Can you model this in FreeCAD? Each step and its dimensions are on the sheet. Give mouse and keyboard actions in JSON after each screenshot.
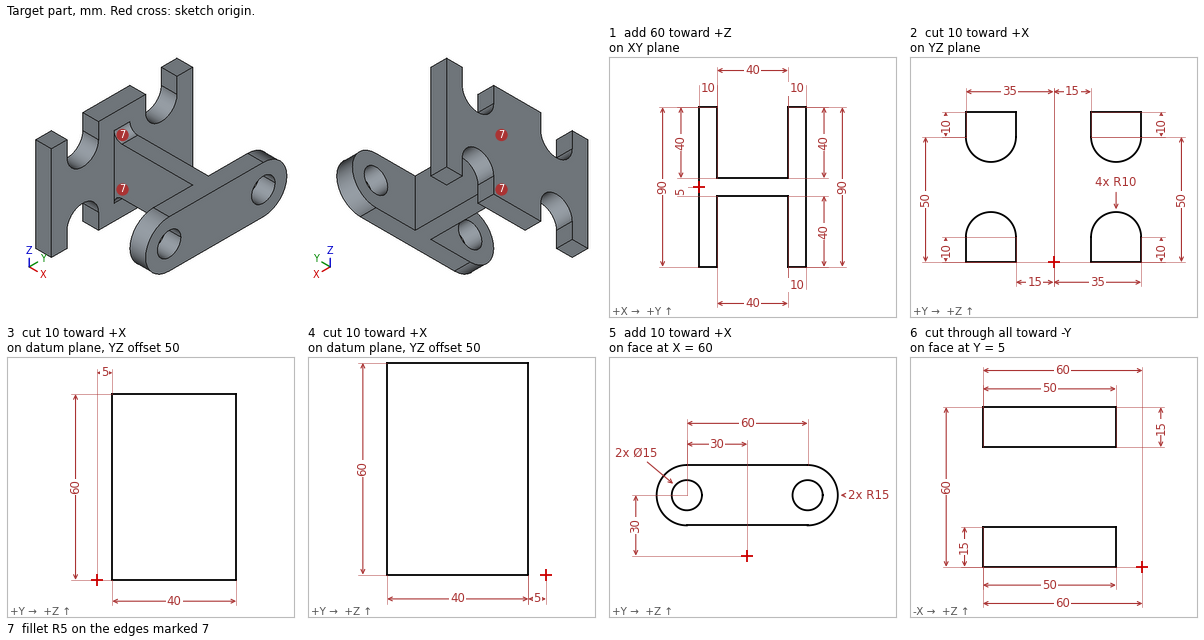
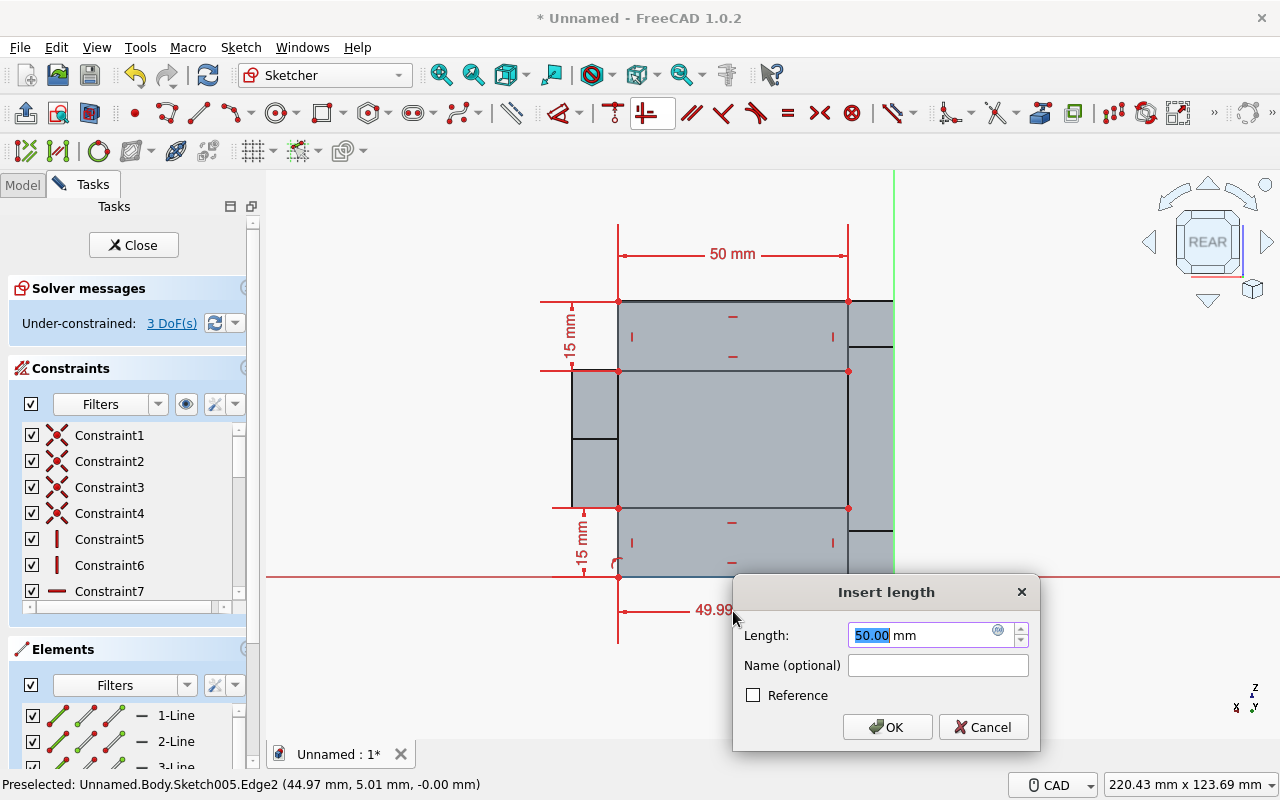
{"action": "type", "text": "50"}
{"action": "key", "text": "Return"}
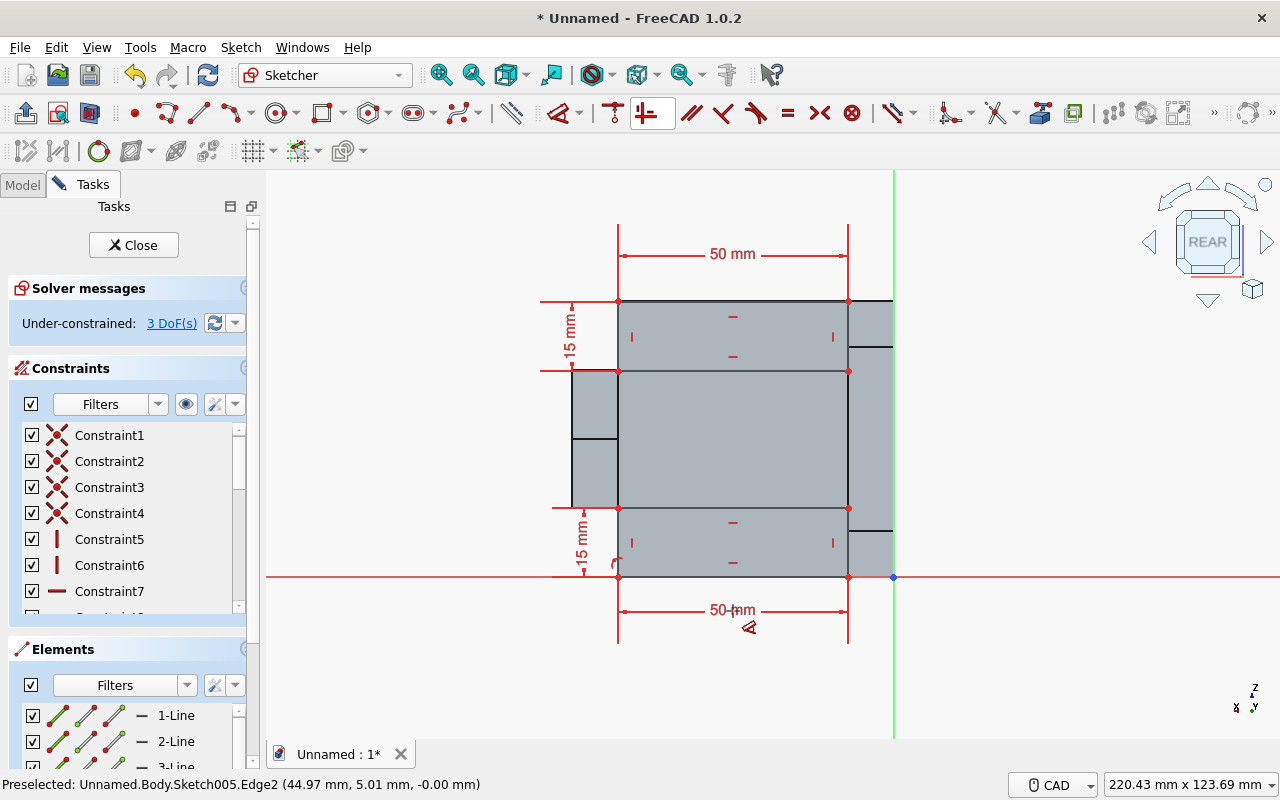
{"action": "left_click", "coordinate": [618, 508]}
{"action": "left_click", "coordinate": [819, 611]}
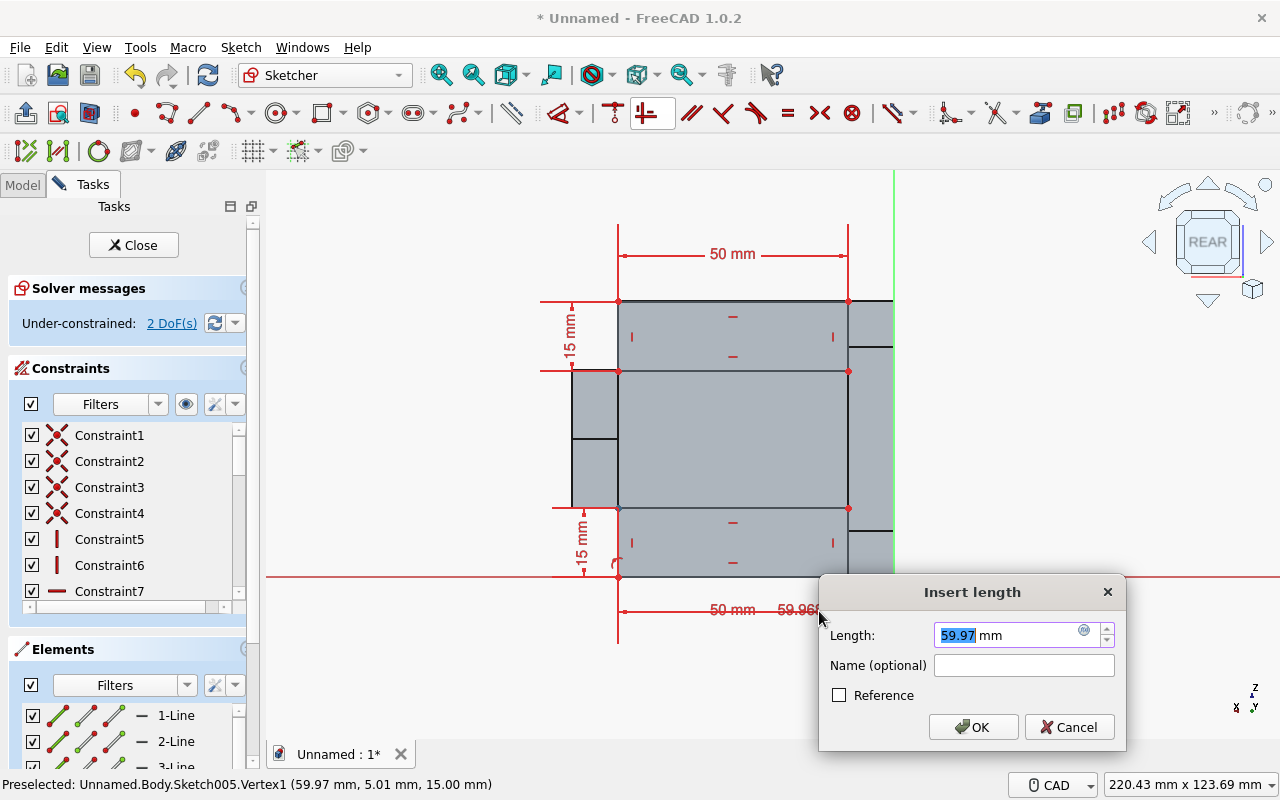
{"action": "type", "text": "60"}
{"action": "key", "text": "Return"}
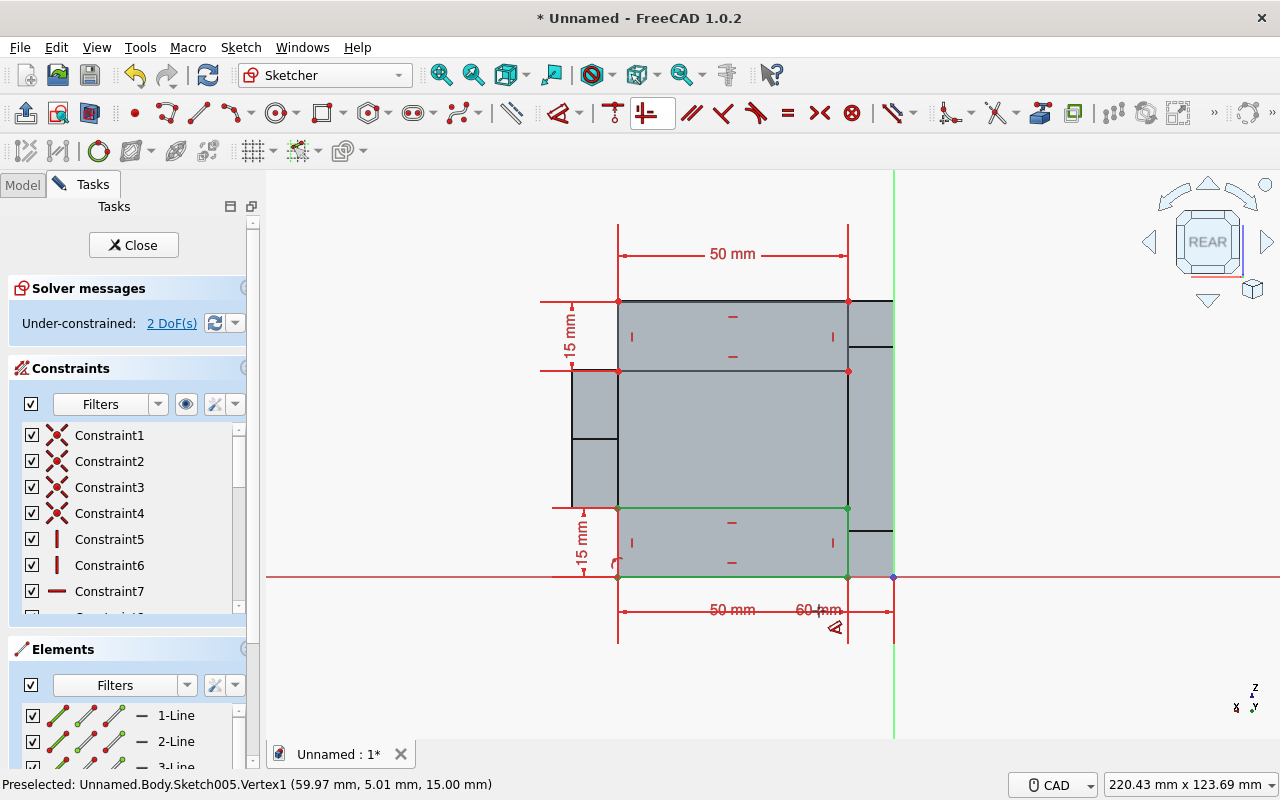
{"action": "left_click", "coordinate": [618, 302]}
{"action": "left_click", "coordinate": [659, 611]}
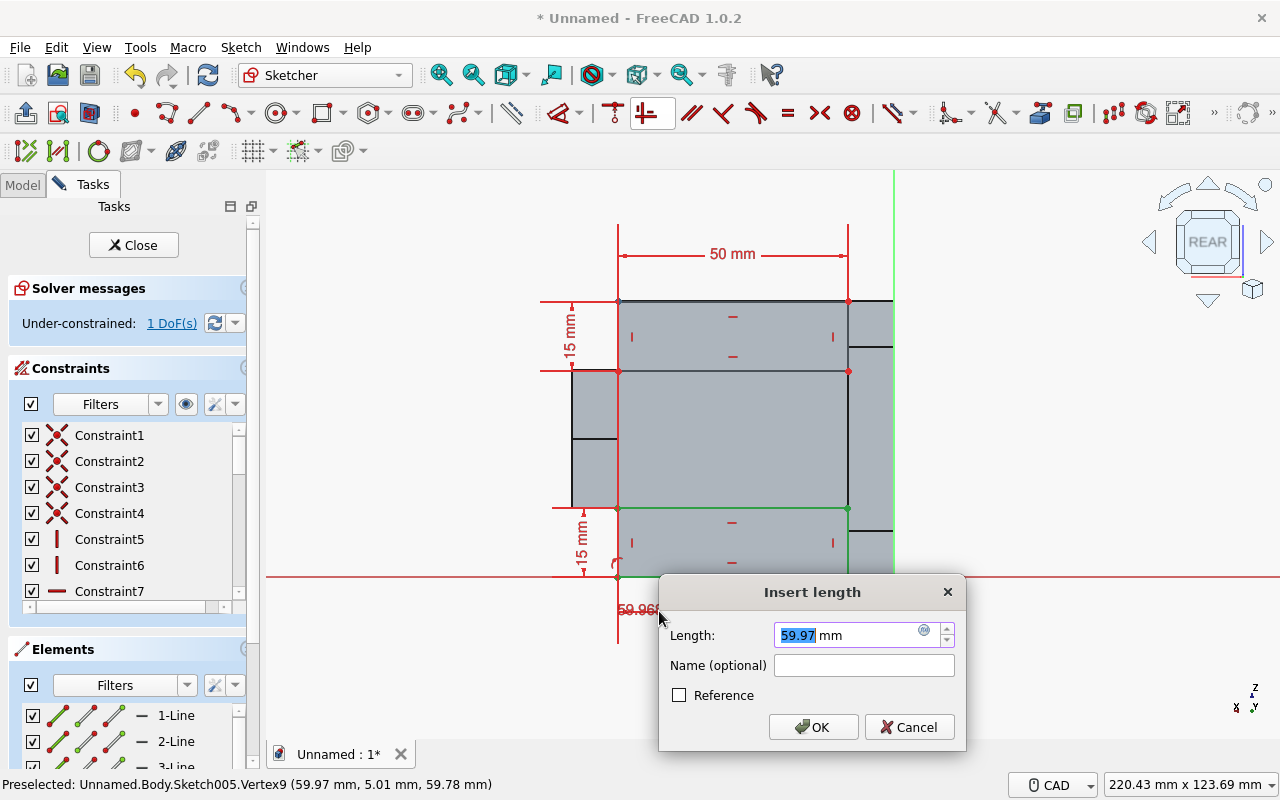
{"action": "type", "text": "60"}
{"action": "key", "text": "Return"}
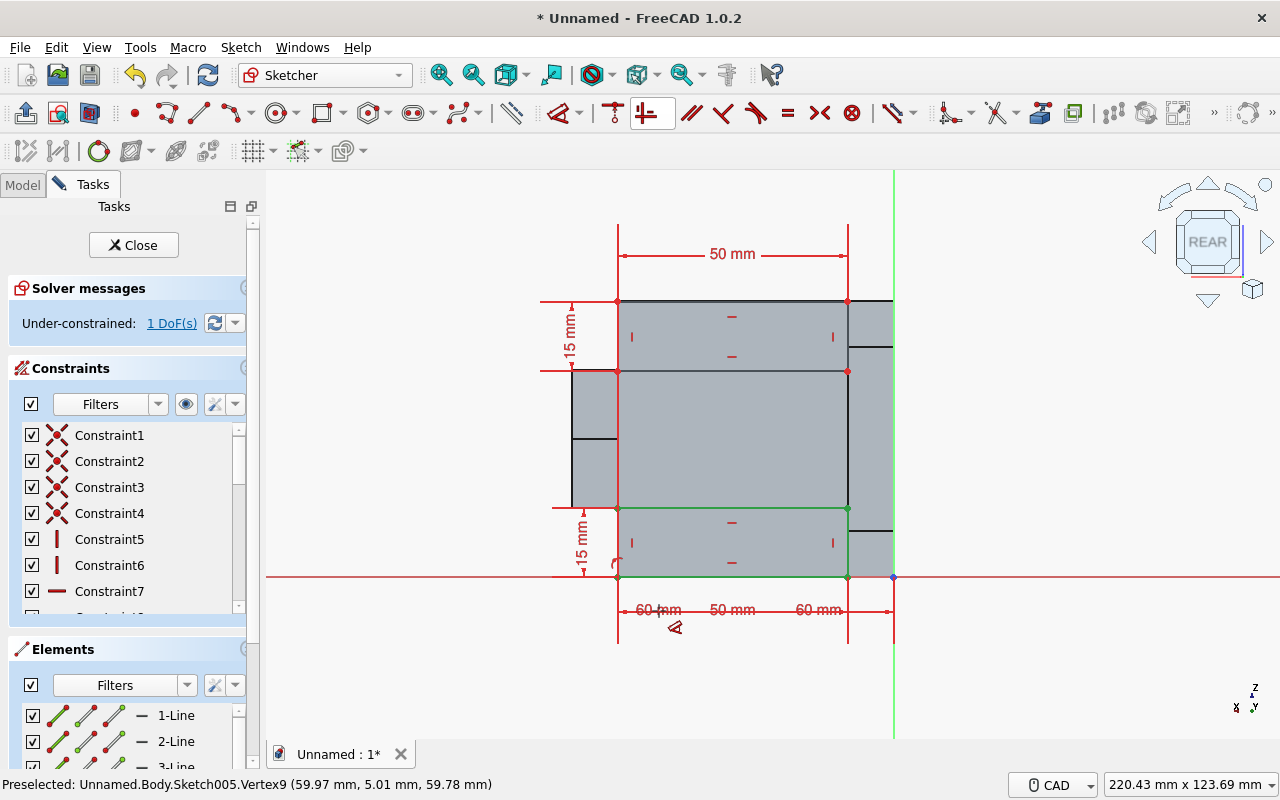
{"action": "left_click", "coordinate": [618, 302]}
{"action": "left_click", "coordinate": [928, 440]}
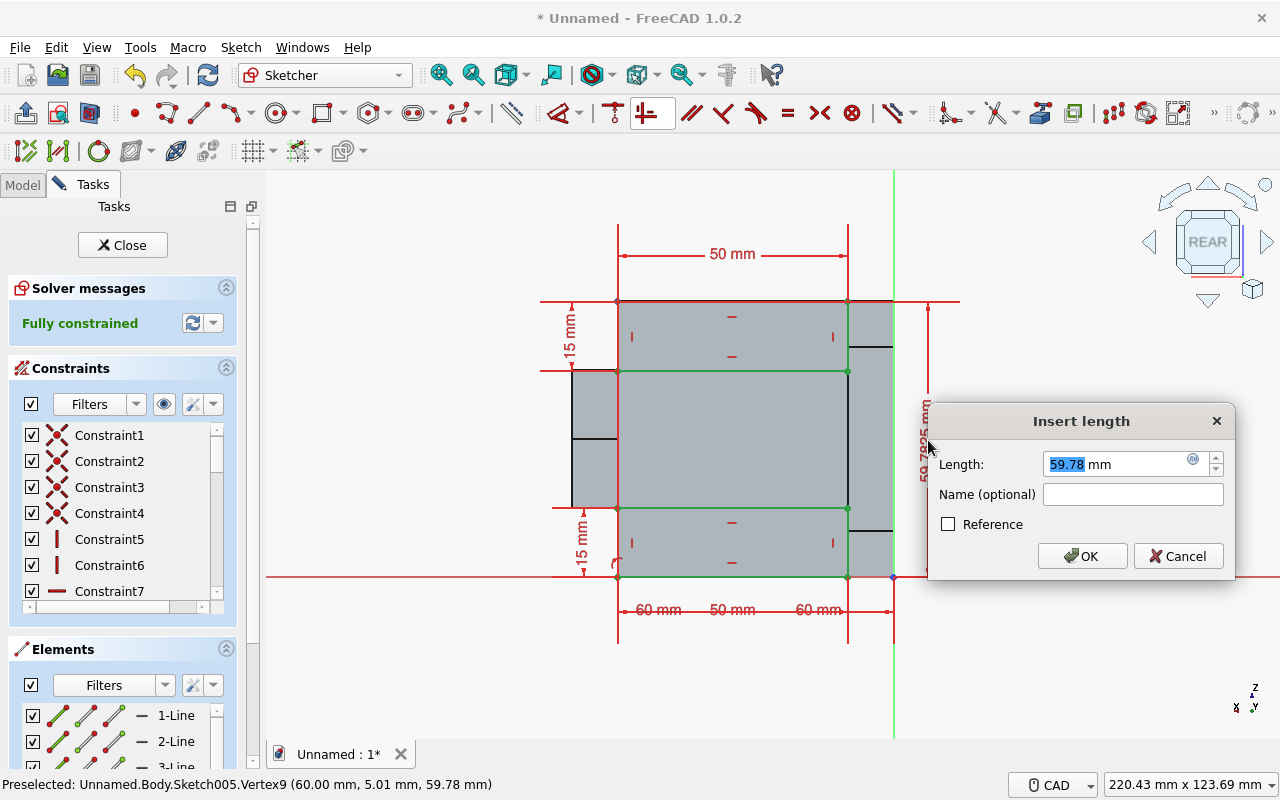
{"action": "type", "text": "60"}
{"action": "key", "text": "Return"}
{"action": "key", "text": "Escape"}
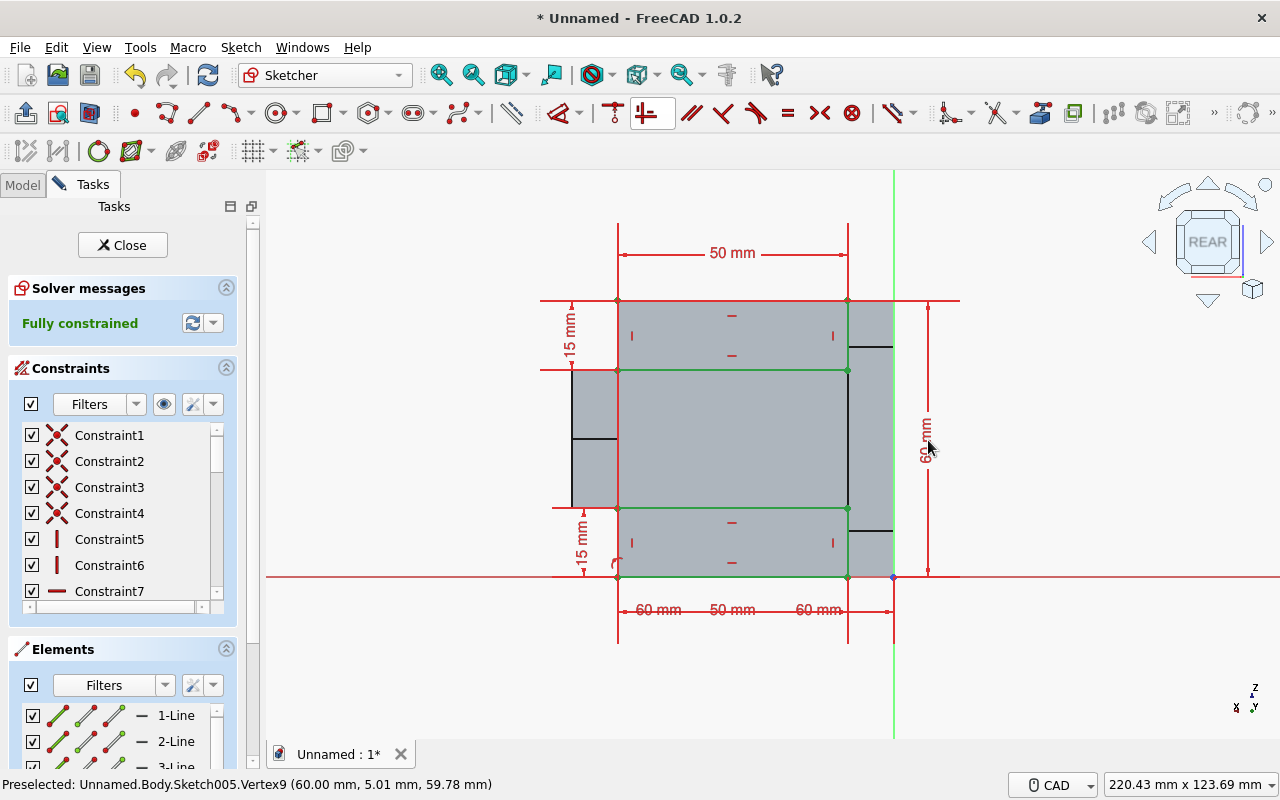
{"action": "left_click", "coordinate": [123, 245]}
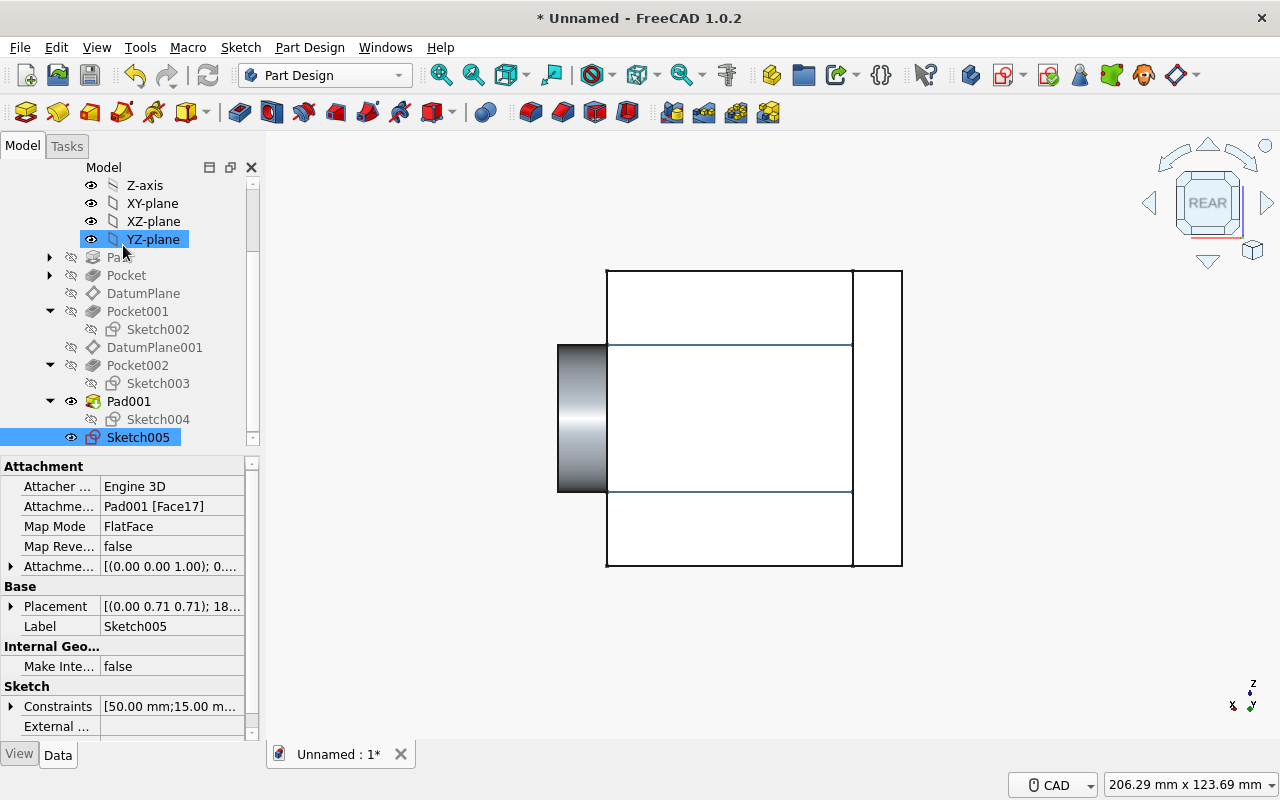
{"action": "left_click", "coordinate": [240, 112]}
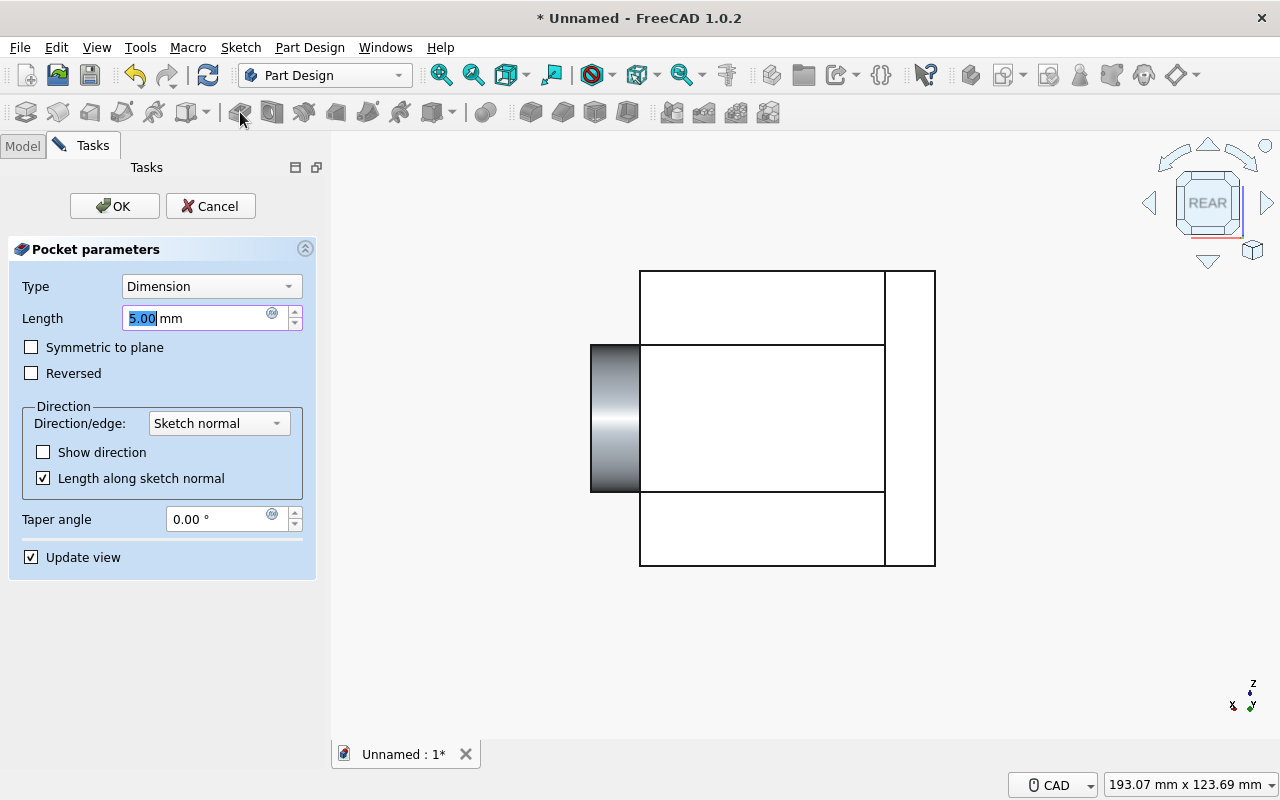
{"action": "left_click", "coordinate": [212, 286]}